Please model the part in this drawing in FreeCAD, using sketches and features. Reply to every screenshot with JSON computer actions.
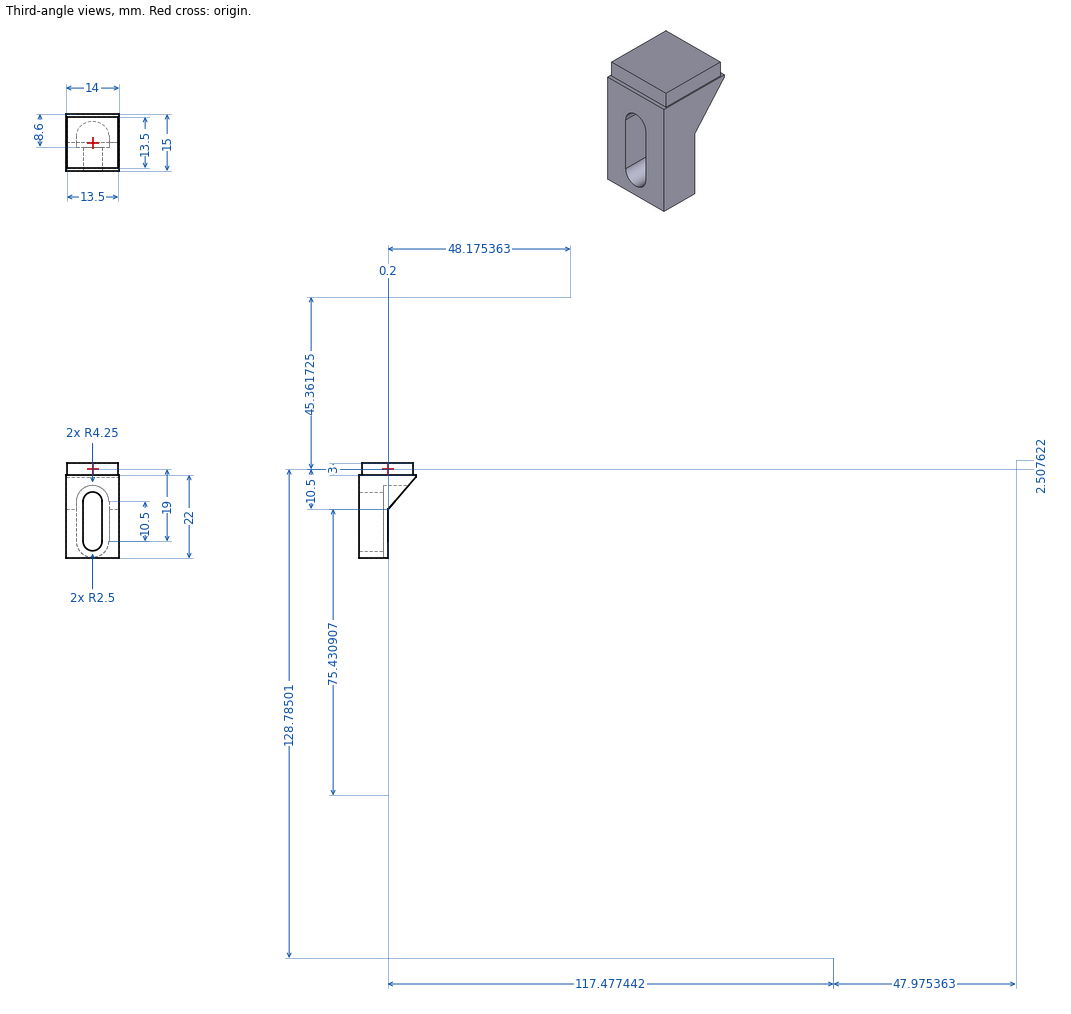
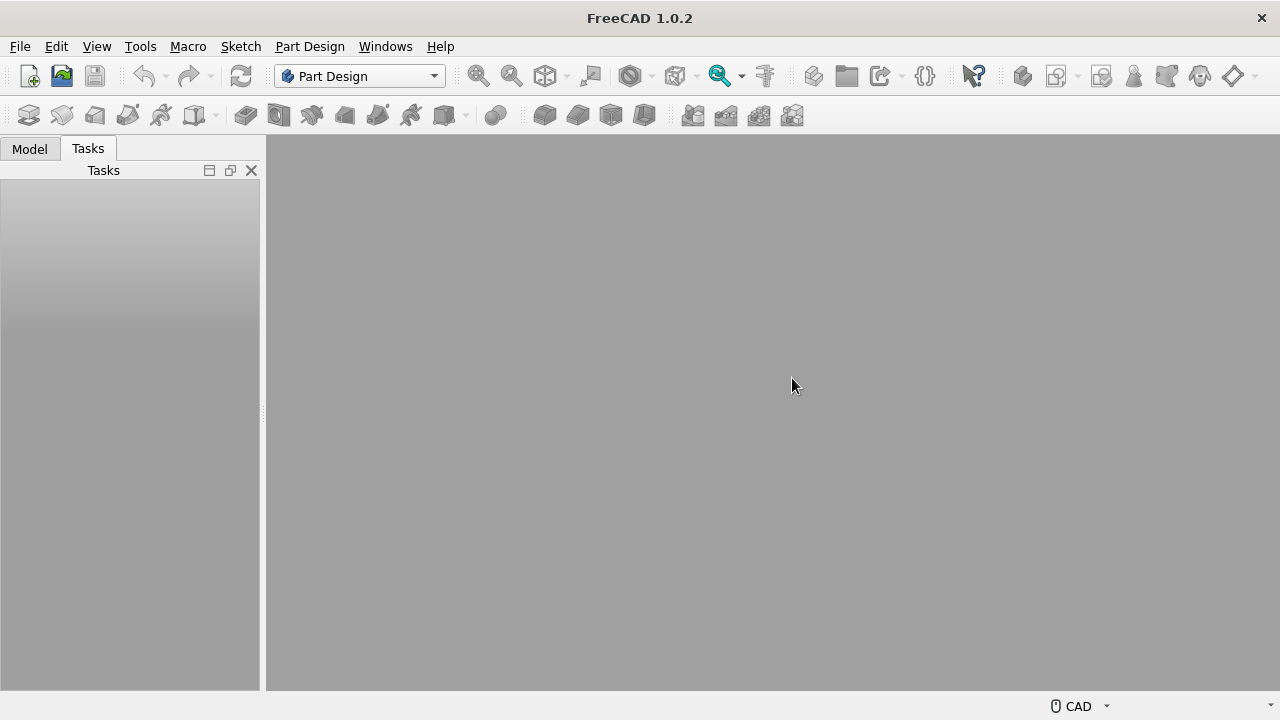
{"action": "key", "text": "ctrl+n"}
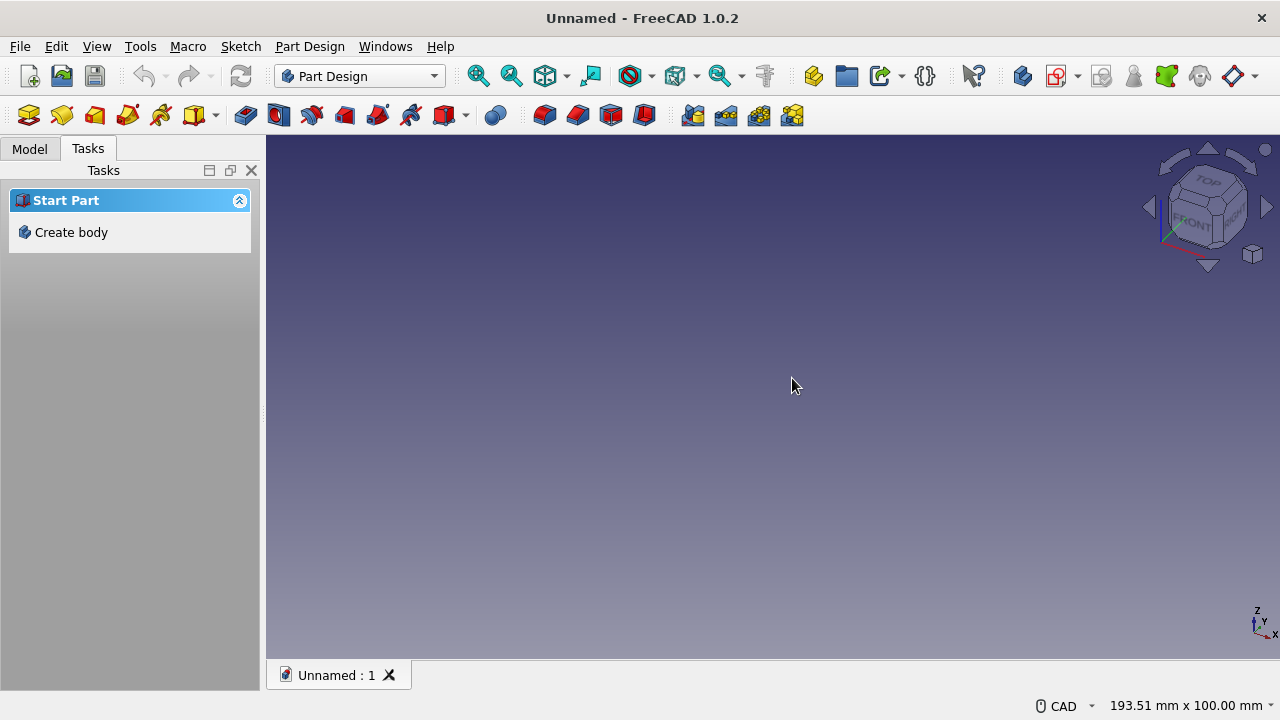
{"action": "left_click", "coordinate": [1056, 76]}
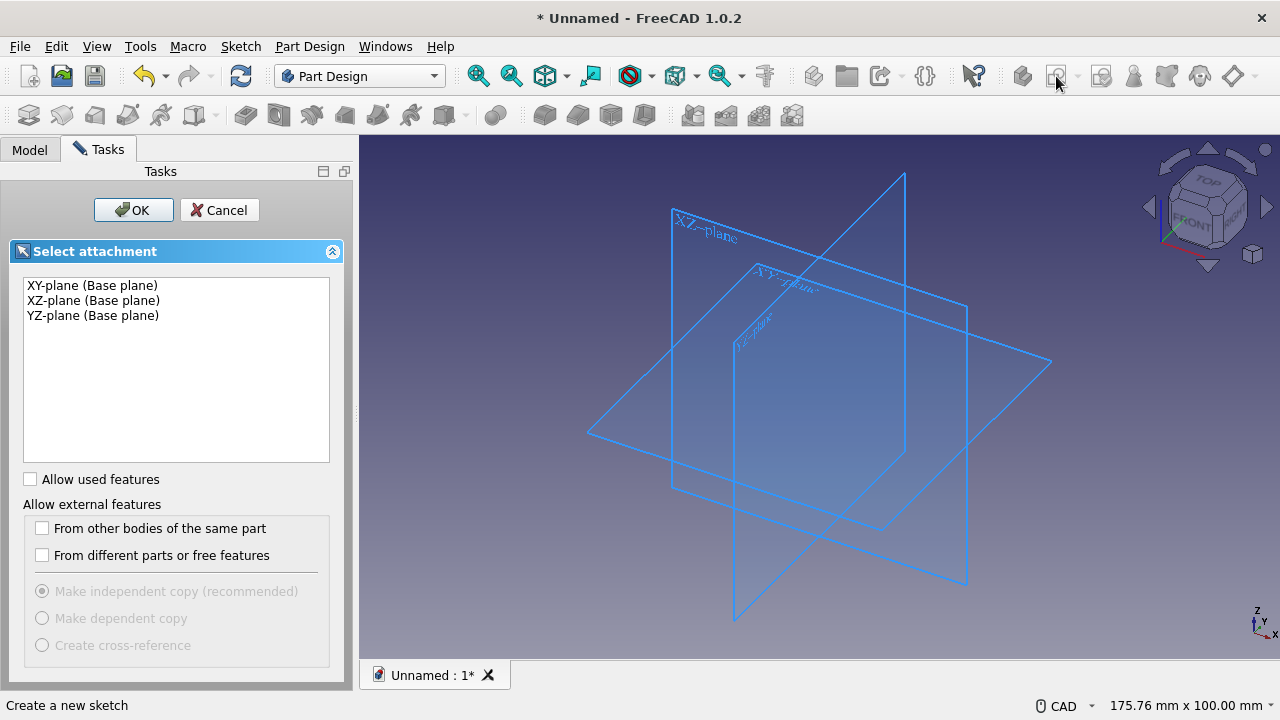
{"action": "left_click", "coordinate": [84, 286]}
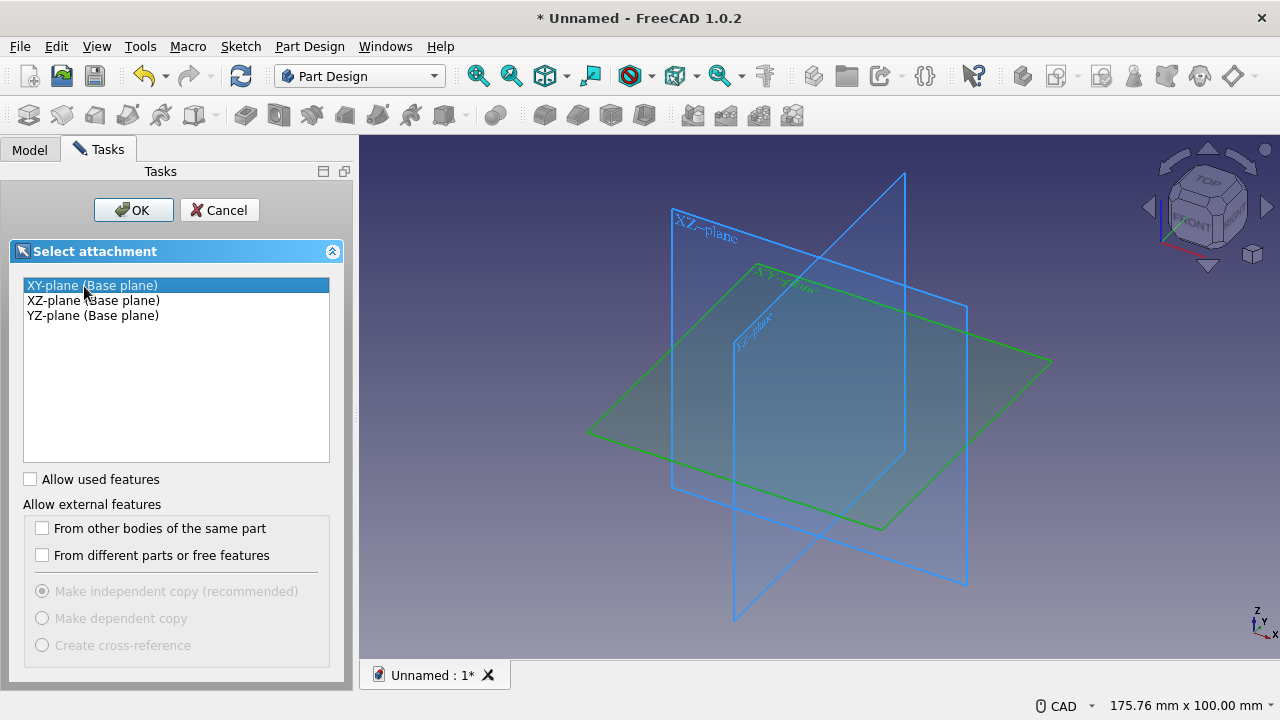
{"action": "left_click", "coordinate": [134, 210]}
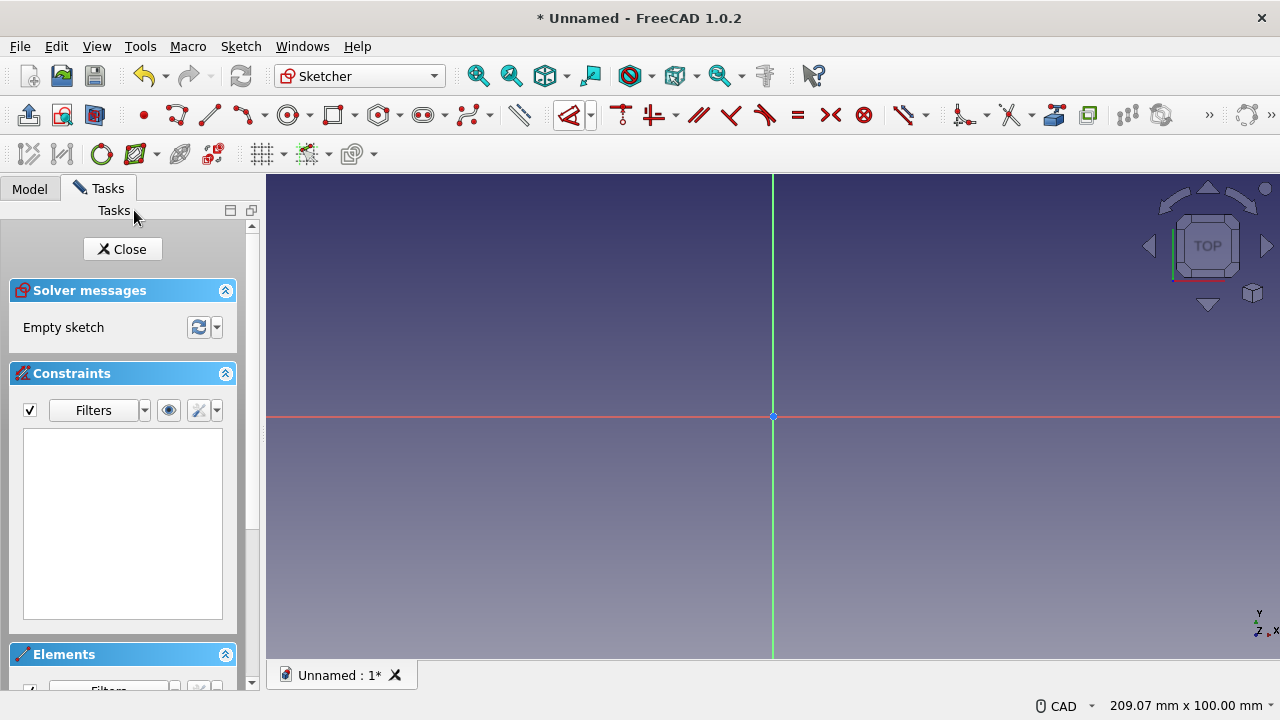
{"action": "scroll", "coordinate": [790, 417], "scroll_direction": "up", "scroll_amount": 8}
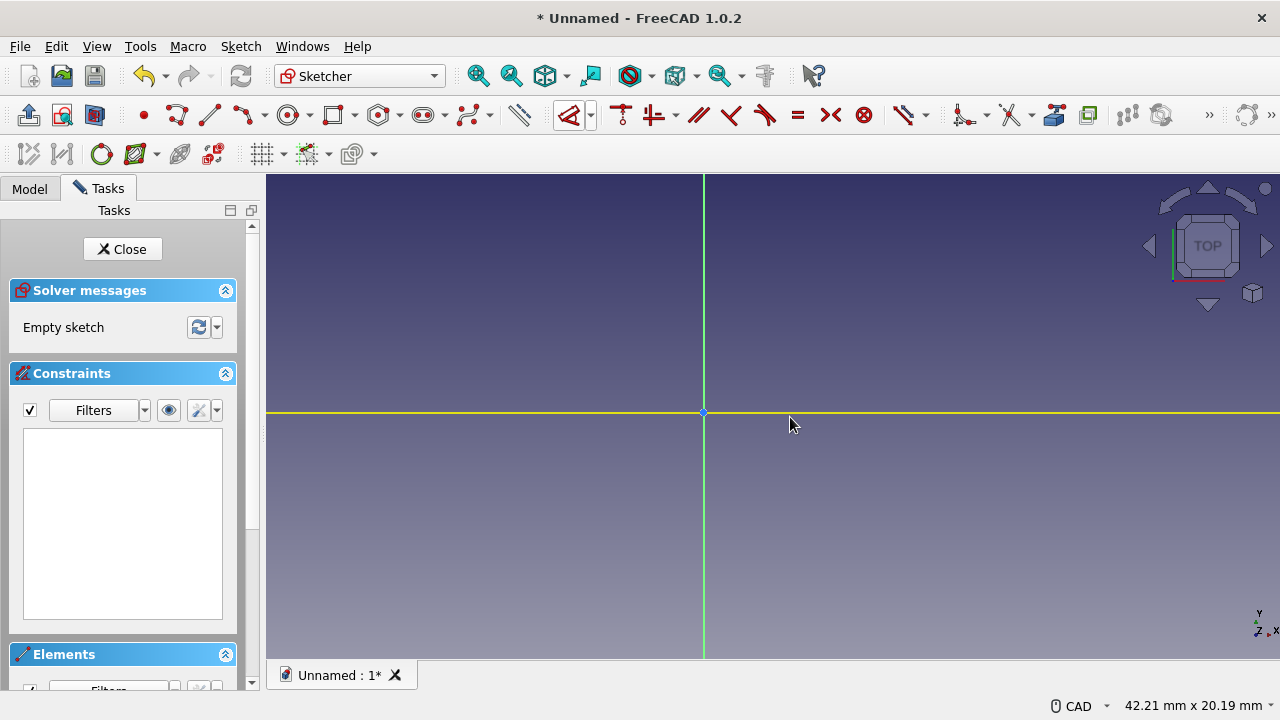
{"action": "key", "text": "g v"}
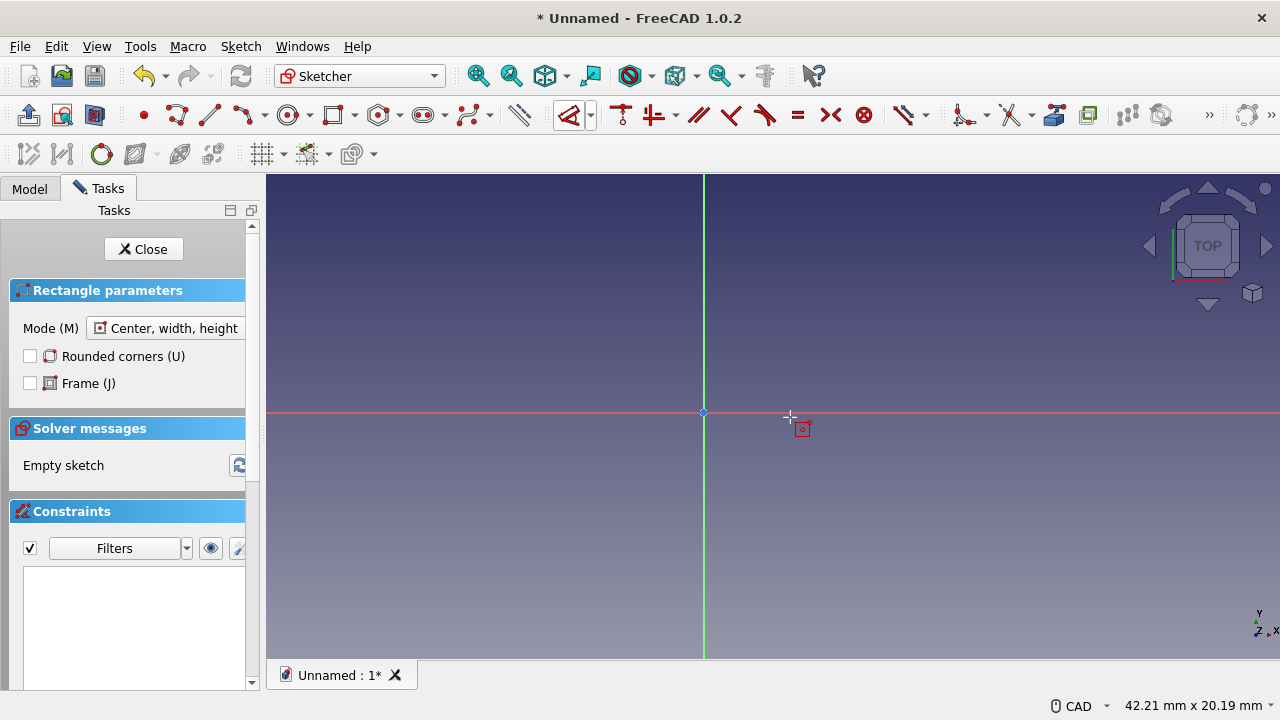
{"action": "left_click", "coordinate": [704, 413]}
{"action": "mouse_move", "coordinate": [866, 250]}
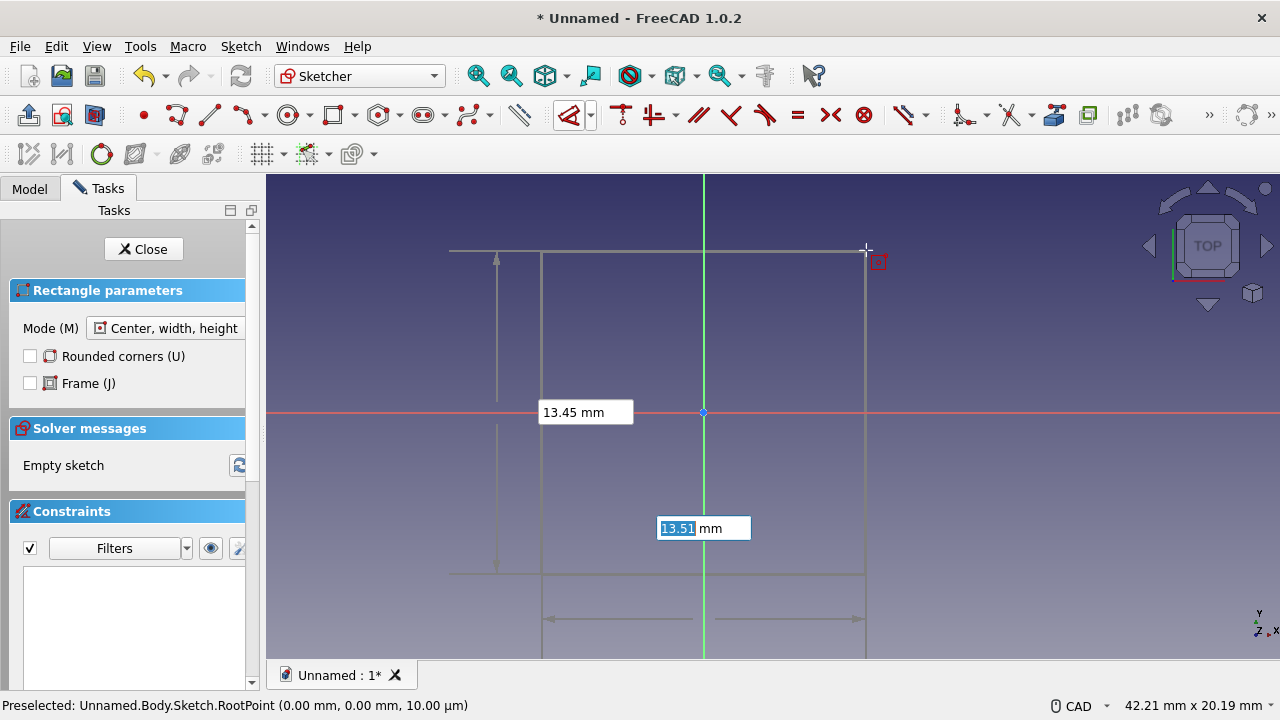
{"action": "type", "text": "13.5"}
{"action": "key", "text": "Tab"}
{"action": "type", "text": "13.5"}
{"action": "key", "text": "Return"}
{"action": "key", "text": "Escape"}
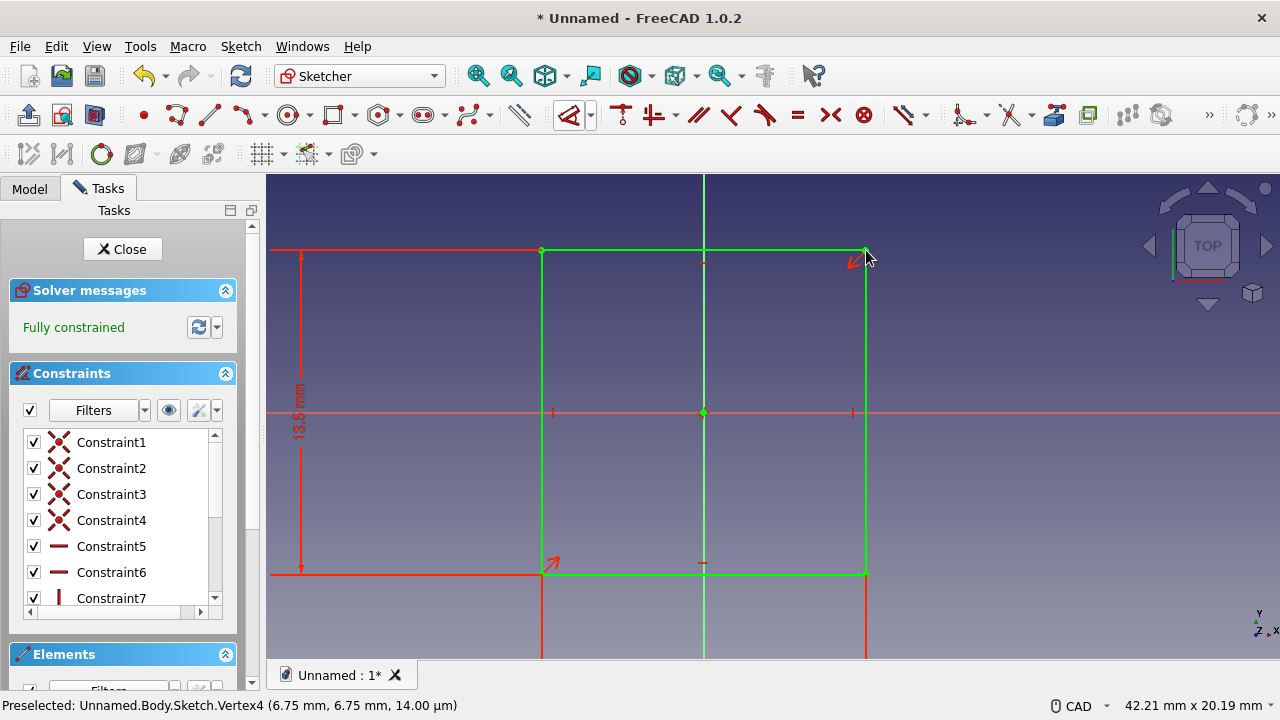
{"action": "left_click", "coordinate": [123, 249]}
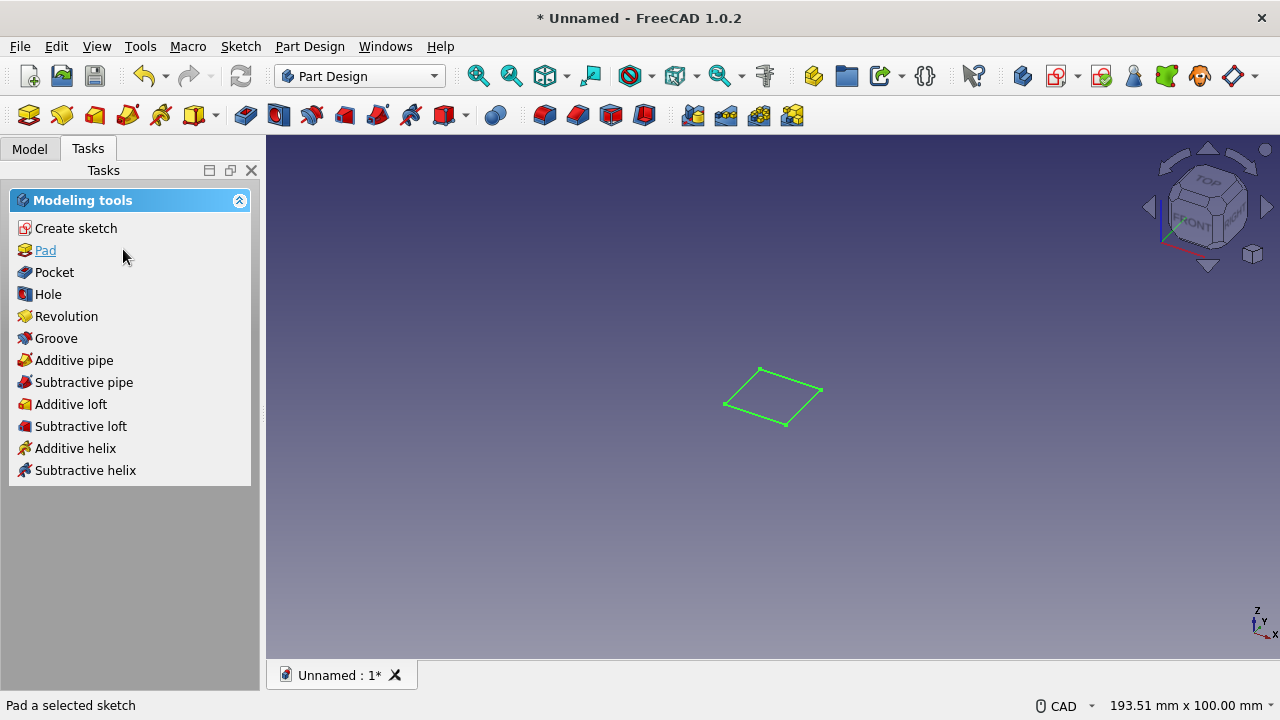
{"action": "left_click", "coordinate": [29, 116]}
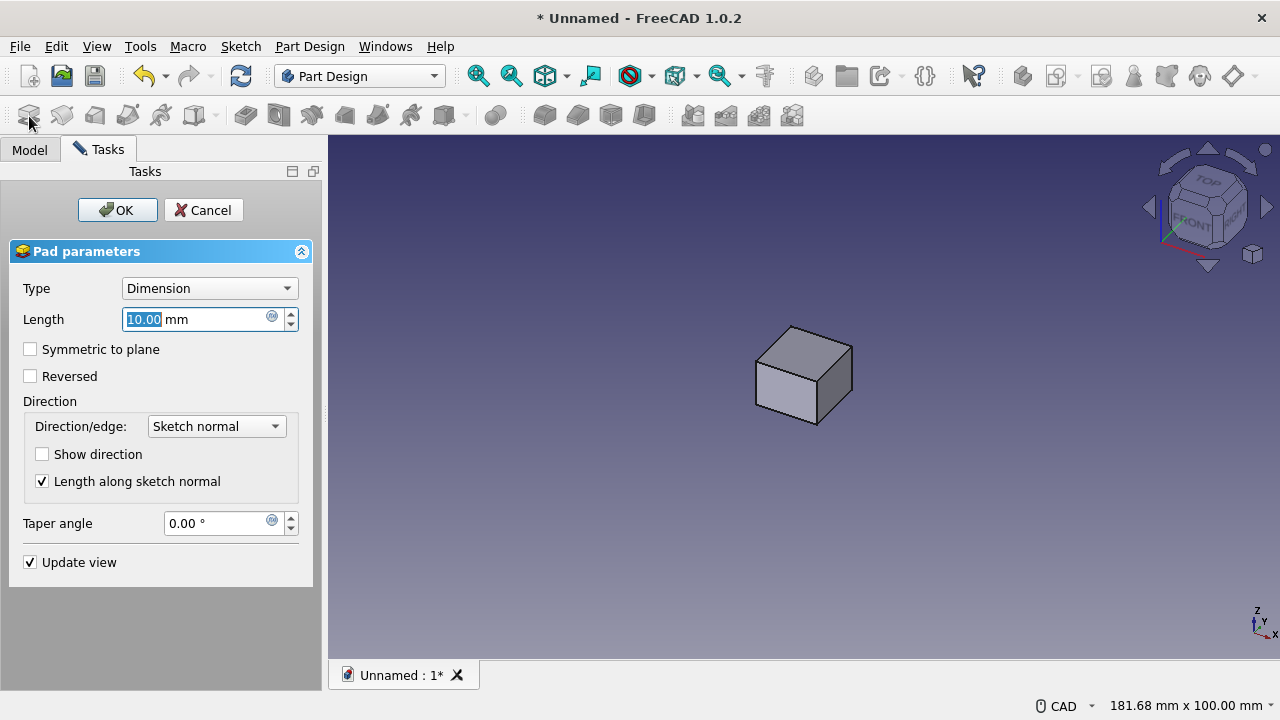
{"action": "type", "text": "3"}
{"action": "key", "text": "Tab"}